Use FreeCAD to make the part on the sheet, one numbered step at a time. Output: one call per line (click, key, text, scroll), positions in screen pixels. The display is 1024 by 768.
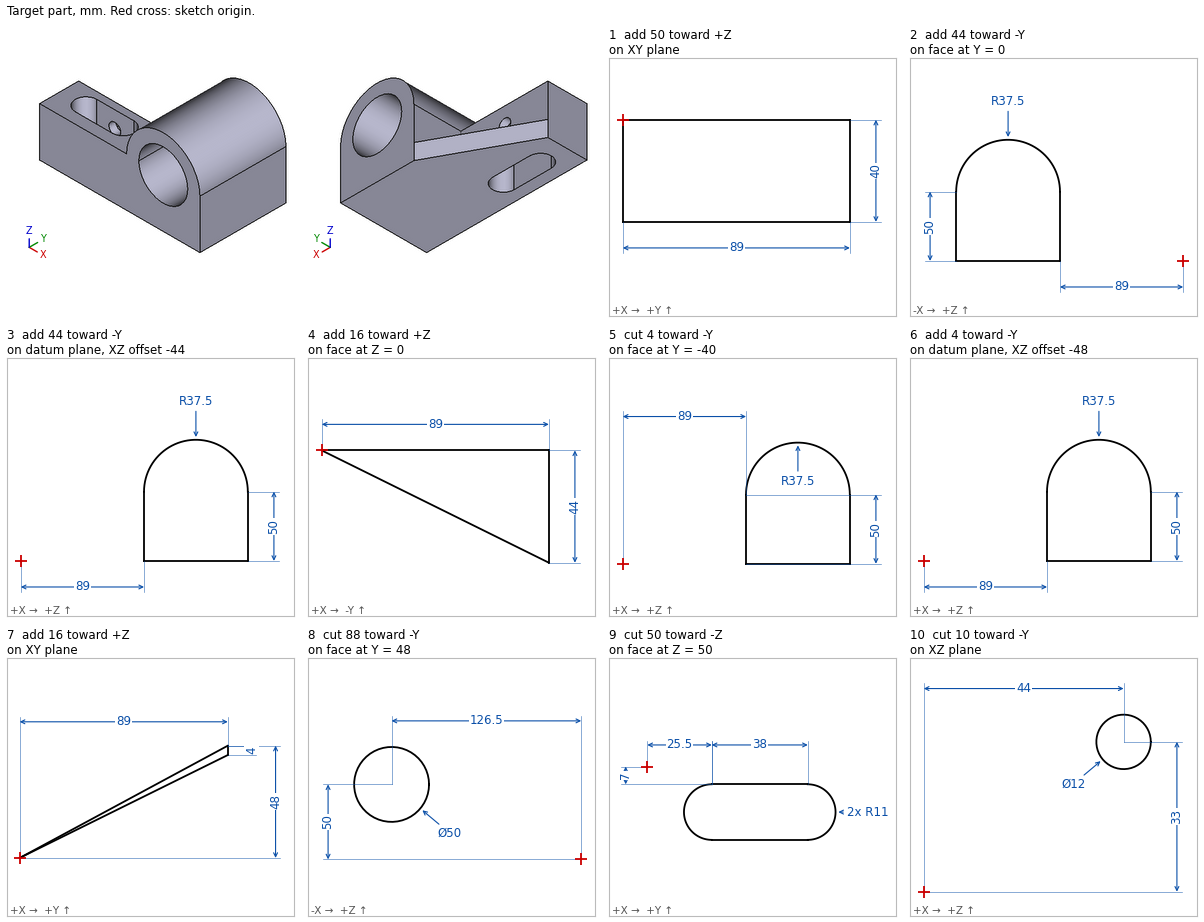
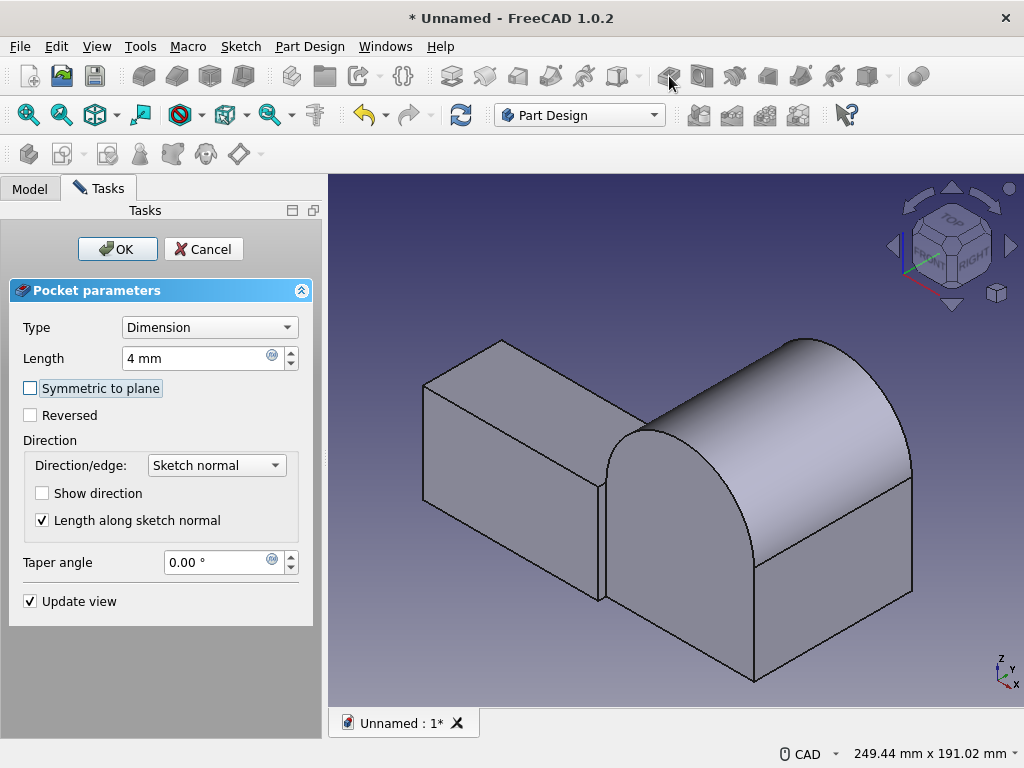
click(31, 415)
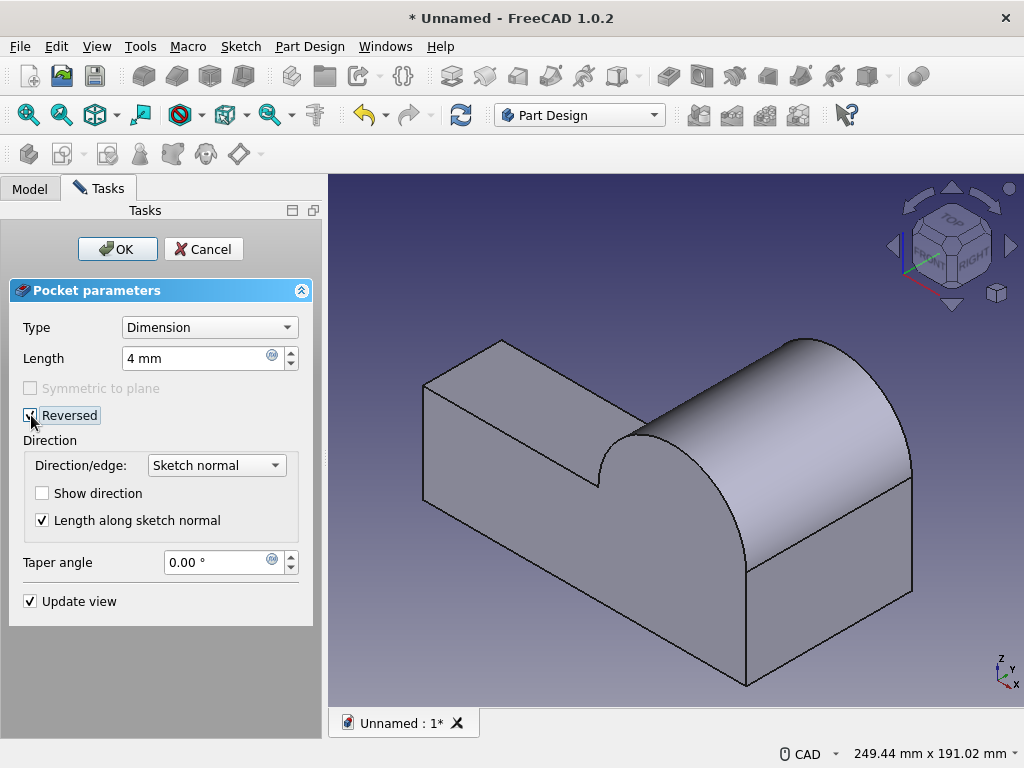
click(118, 249)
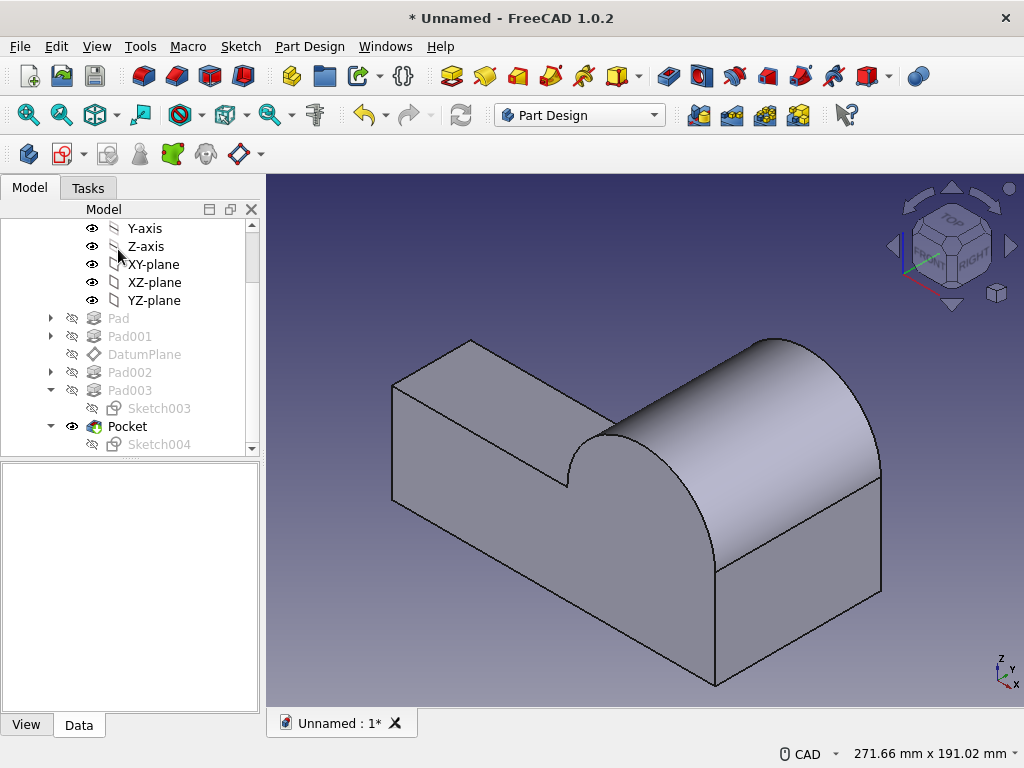
scroll(161, 332, down, 3)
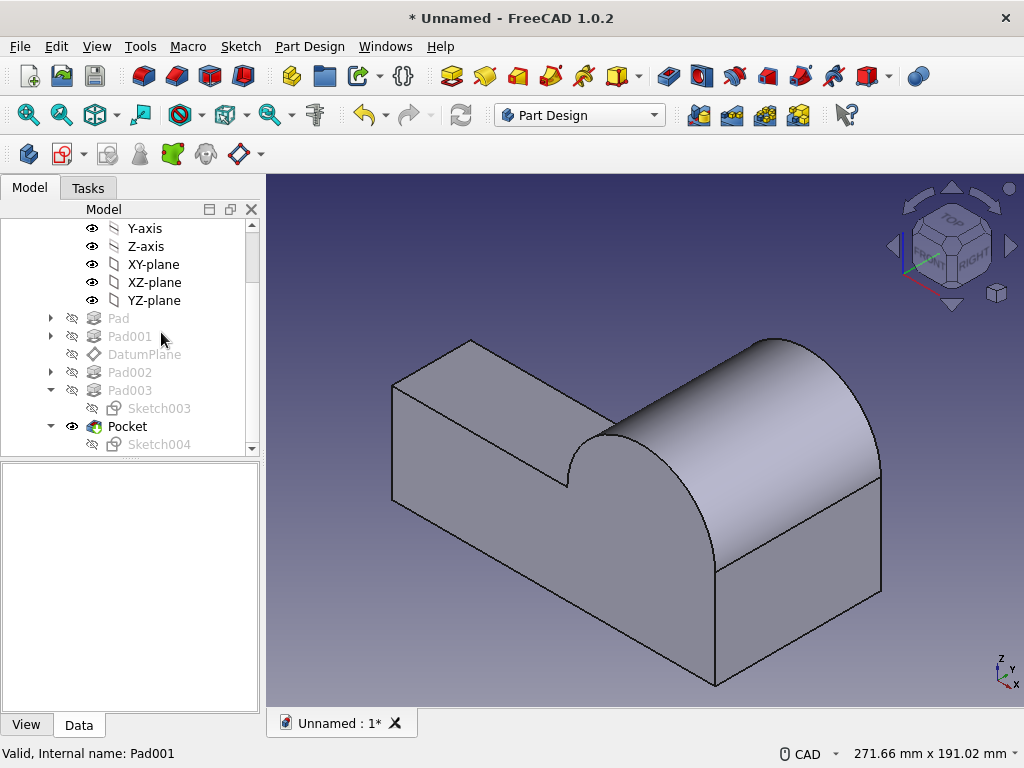
scroll(161, 332, up, 15)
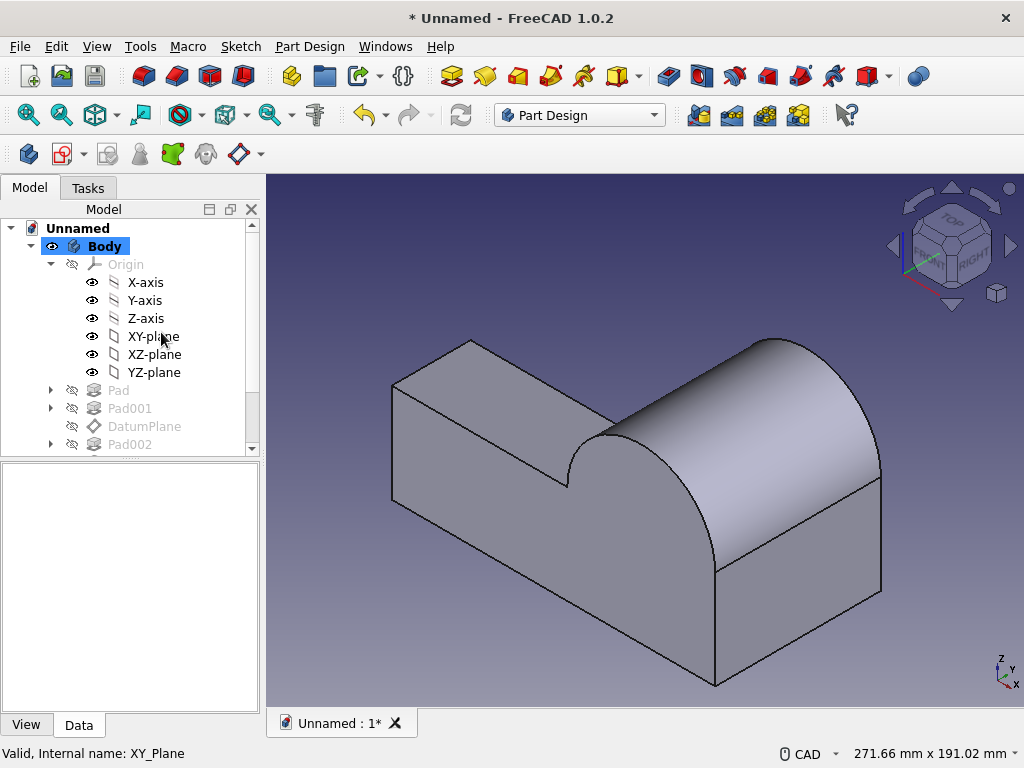
click(137, 354)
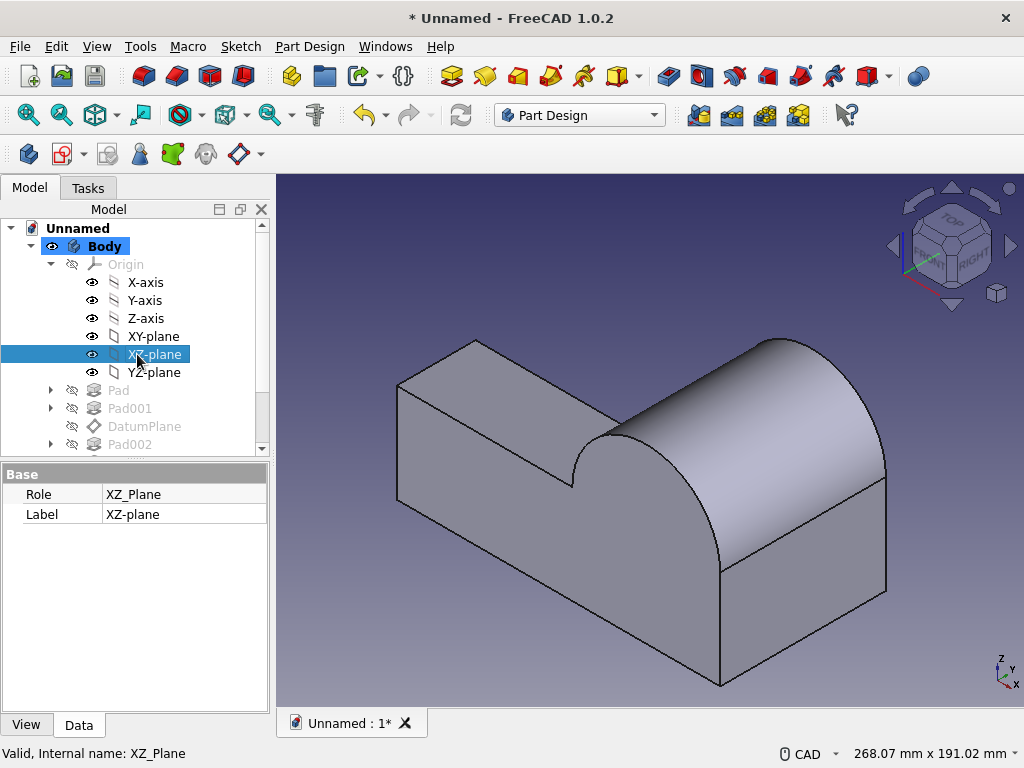
click(238, 154)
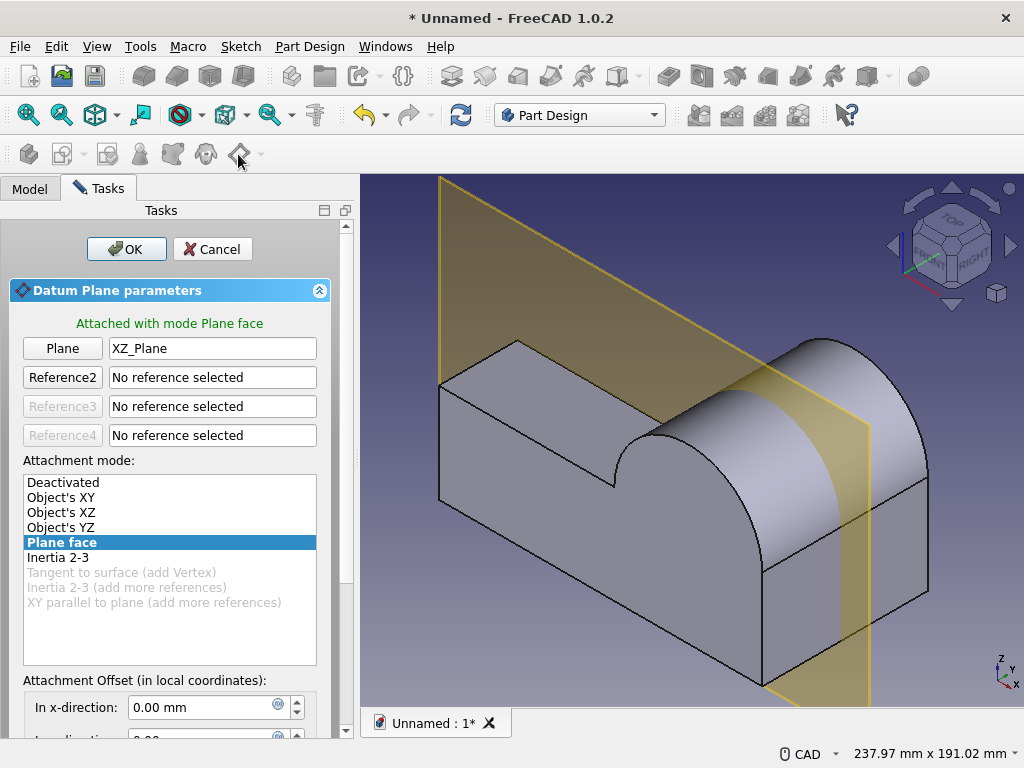
scroll(346, 479, down, 2)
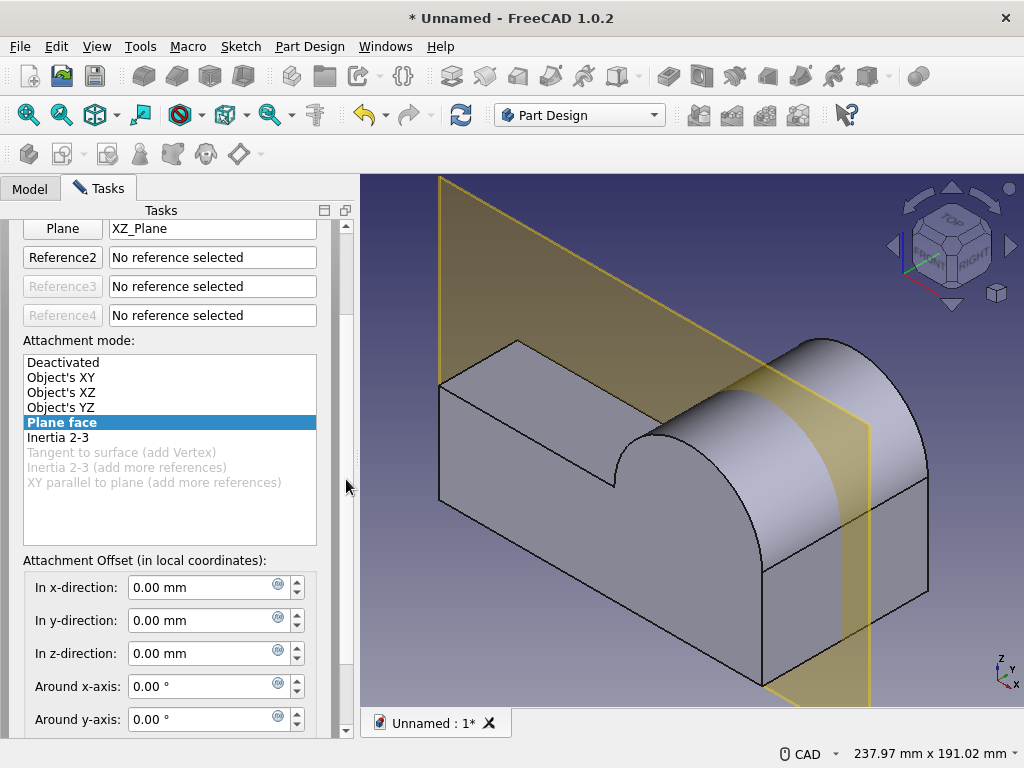
triple_click(210, 654)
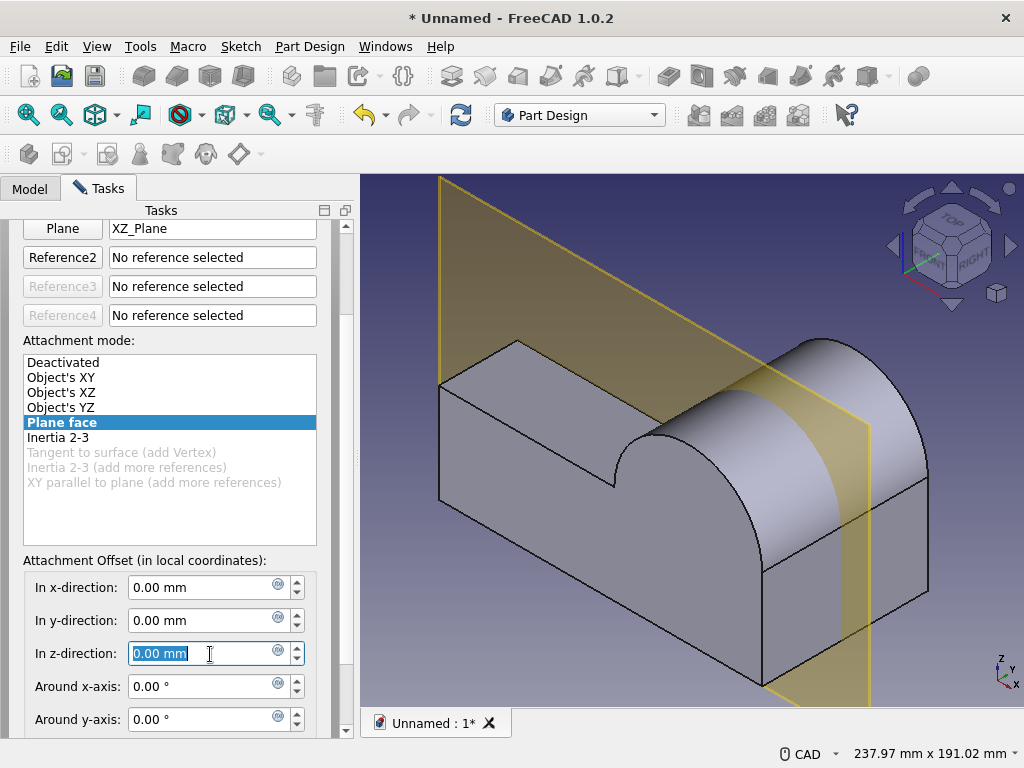
text(-48)
key(Tab)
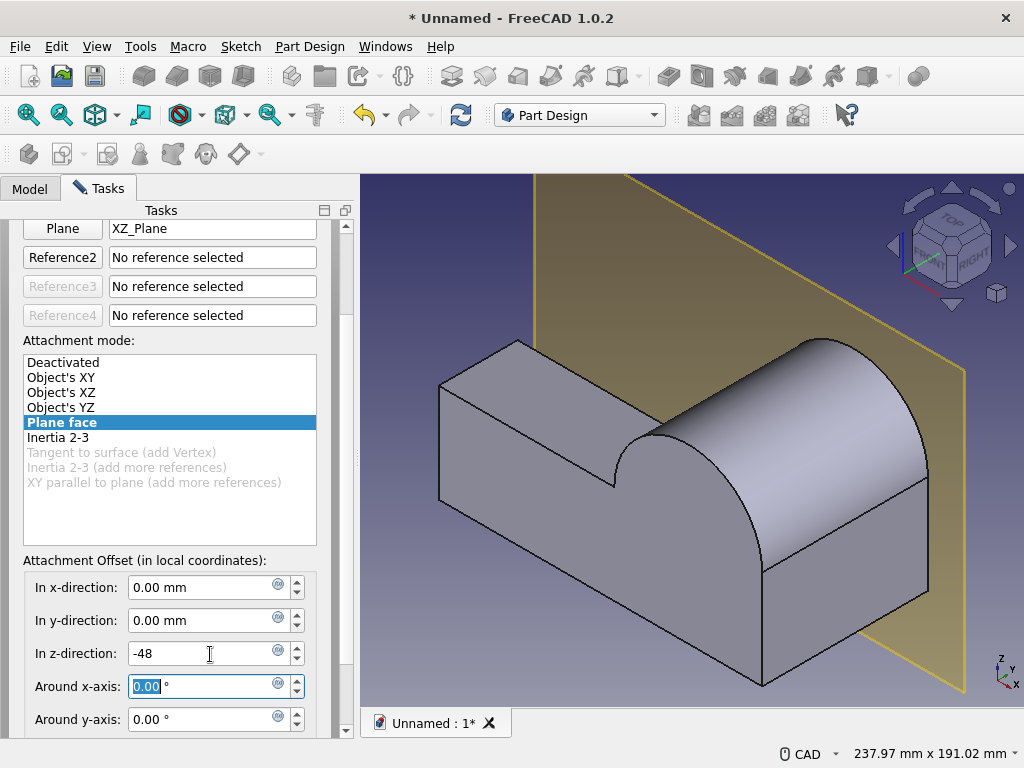
scroll(346, 479, up, 3)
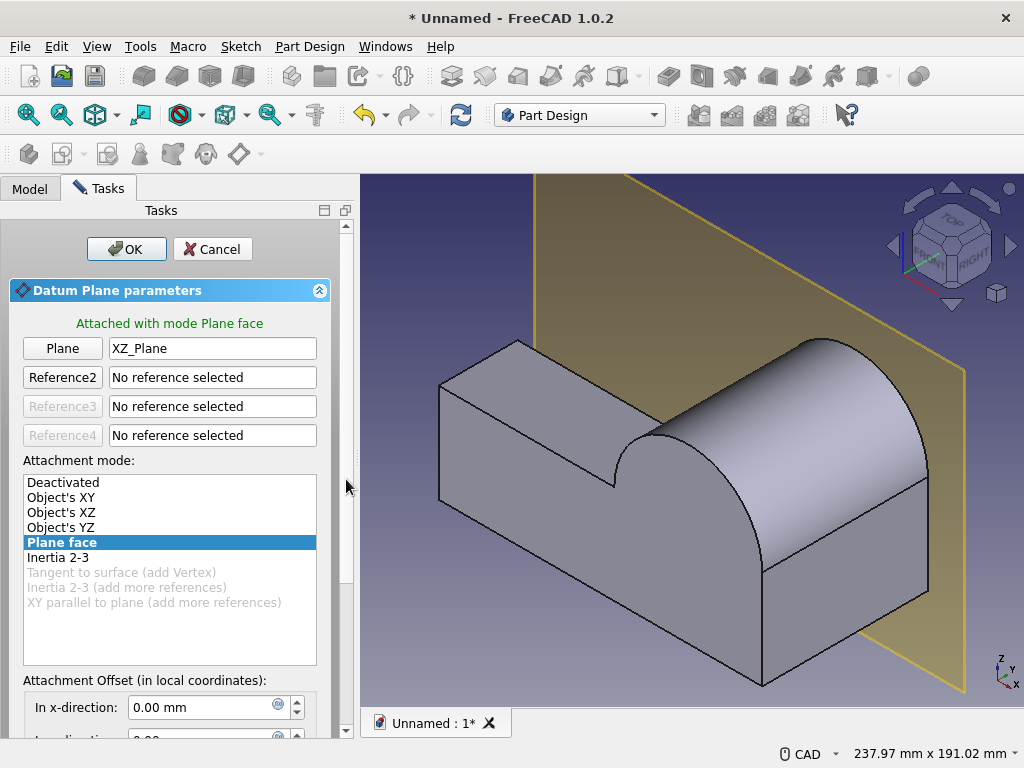
click(127, 249)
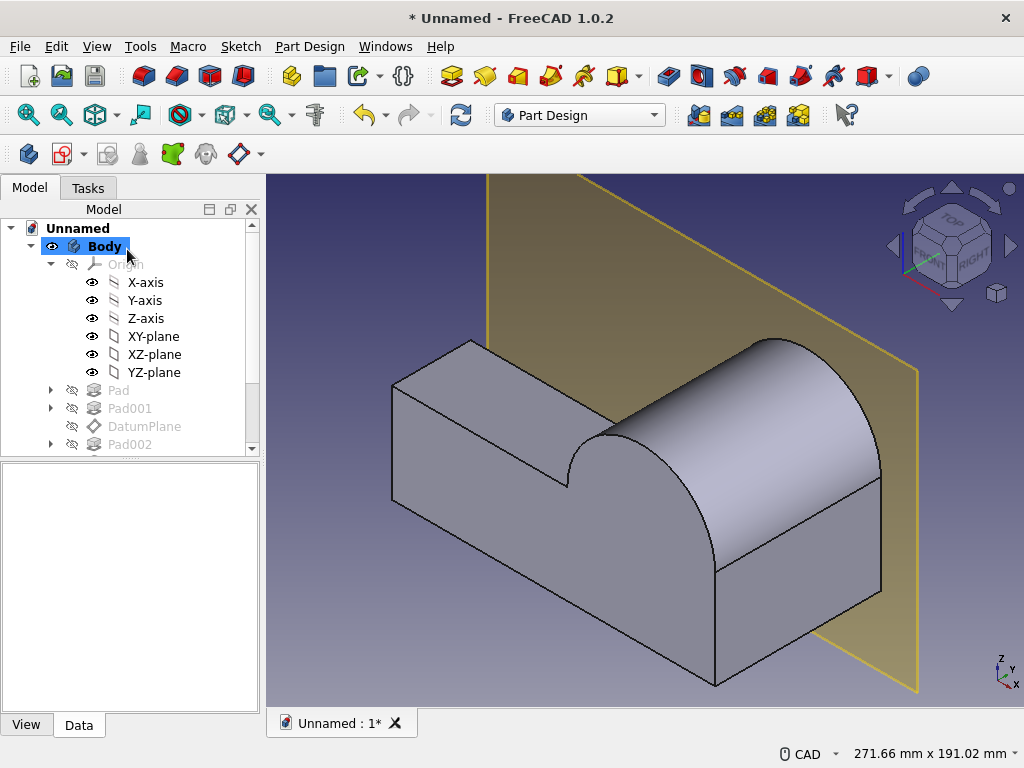
scroll(101, 332, down, 3)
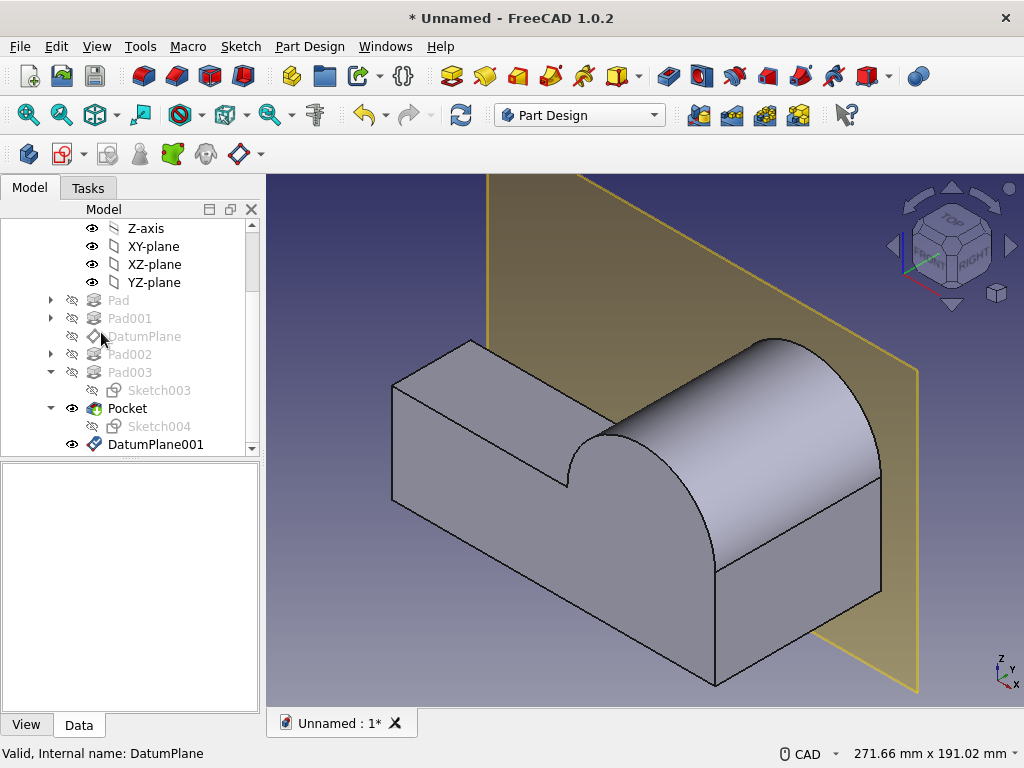
click(117, 444)